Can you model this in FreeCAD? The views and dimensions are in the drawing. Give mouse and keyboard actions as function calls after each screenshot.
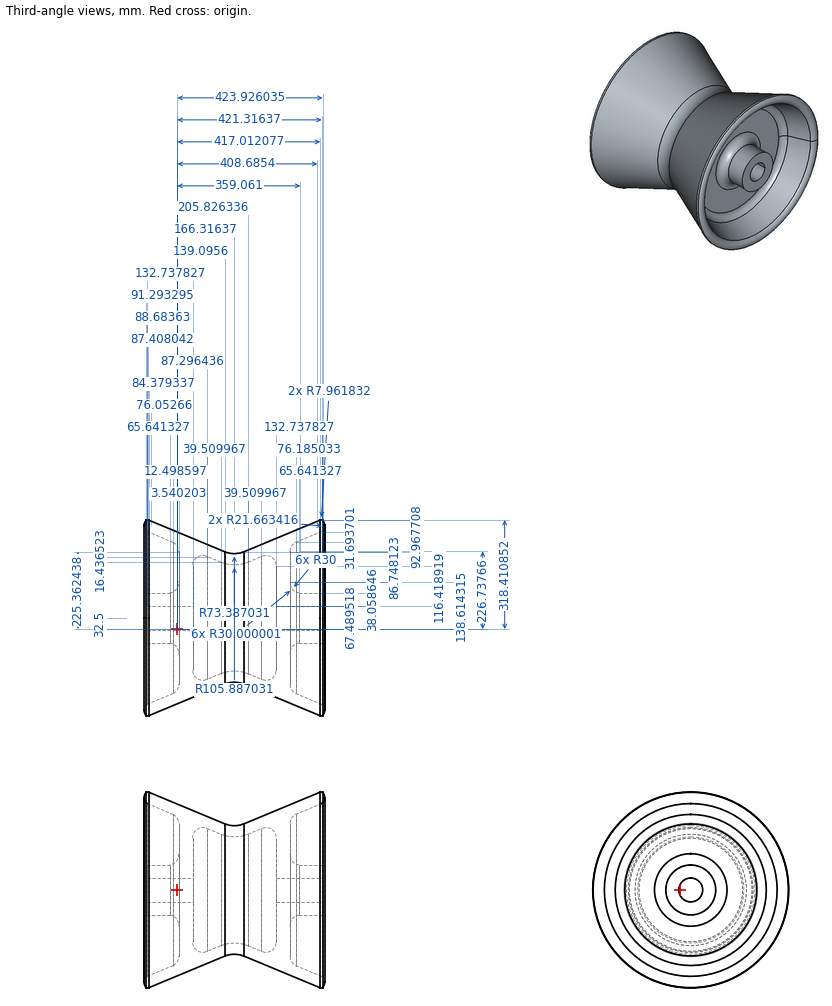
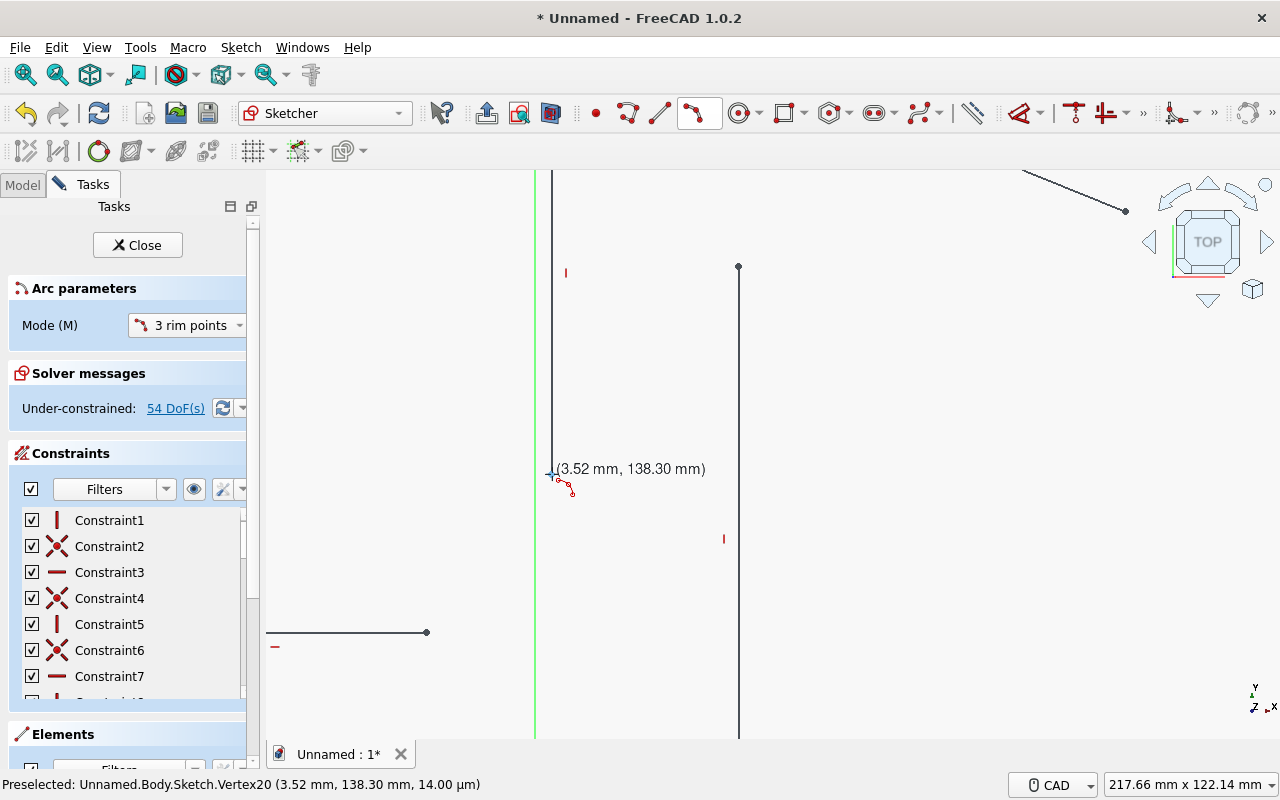
scroll(551, 474, down, 8)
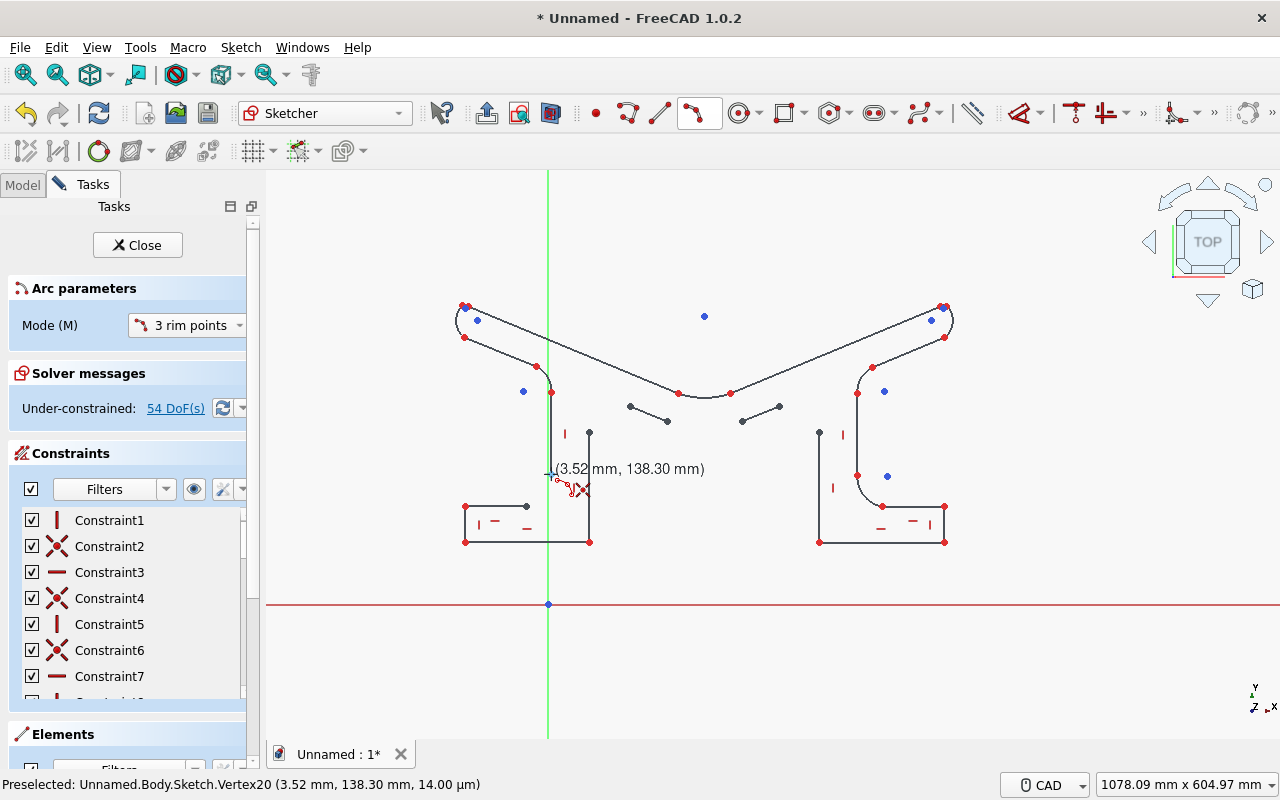
click(526, 506)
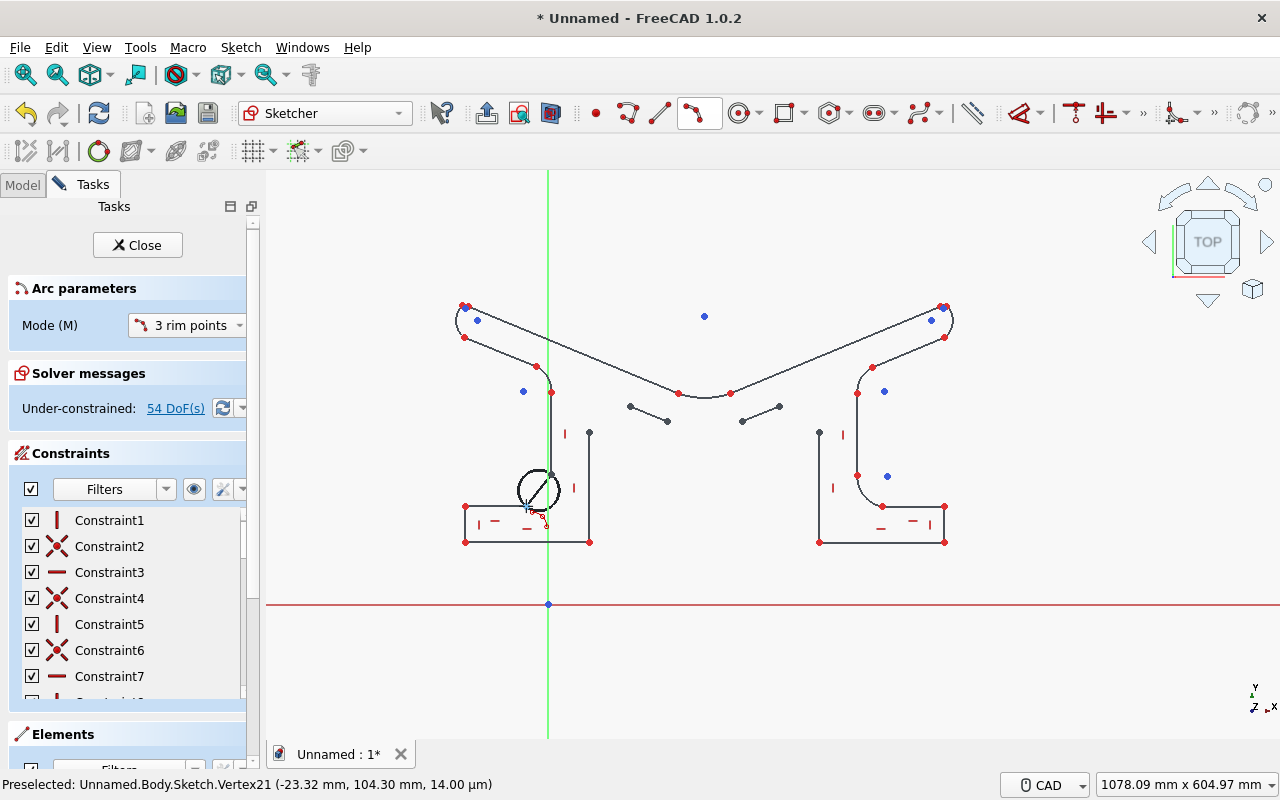
scroll(539, 501, up, 5)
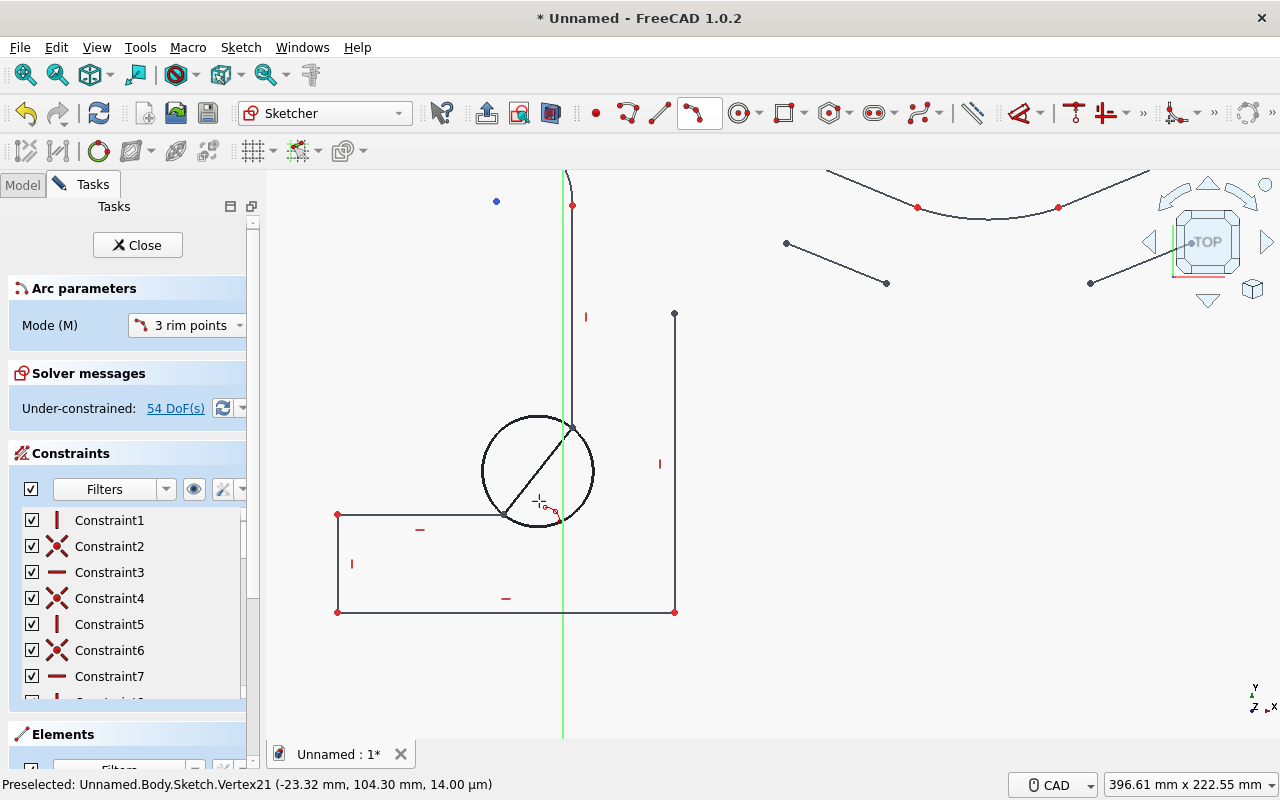
click(538, 500)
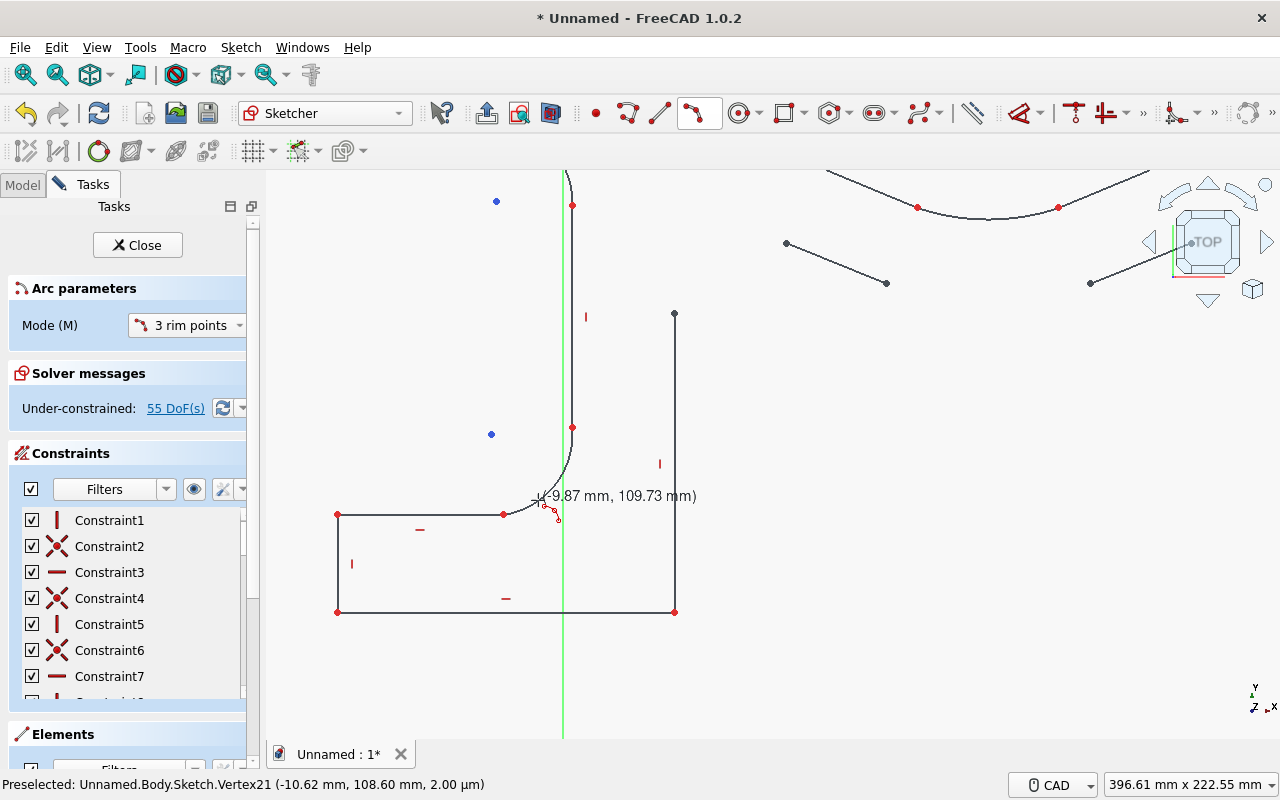
click(675, 314)
click(786, 243)
click(711, 244)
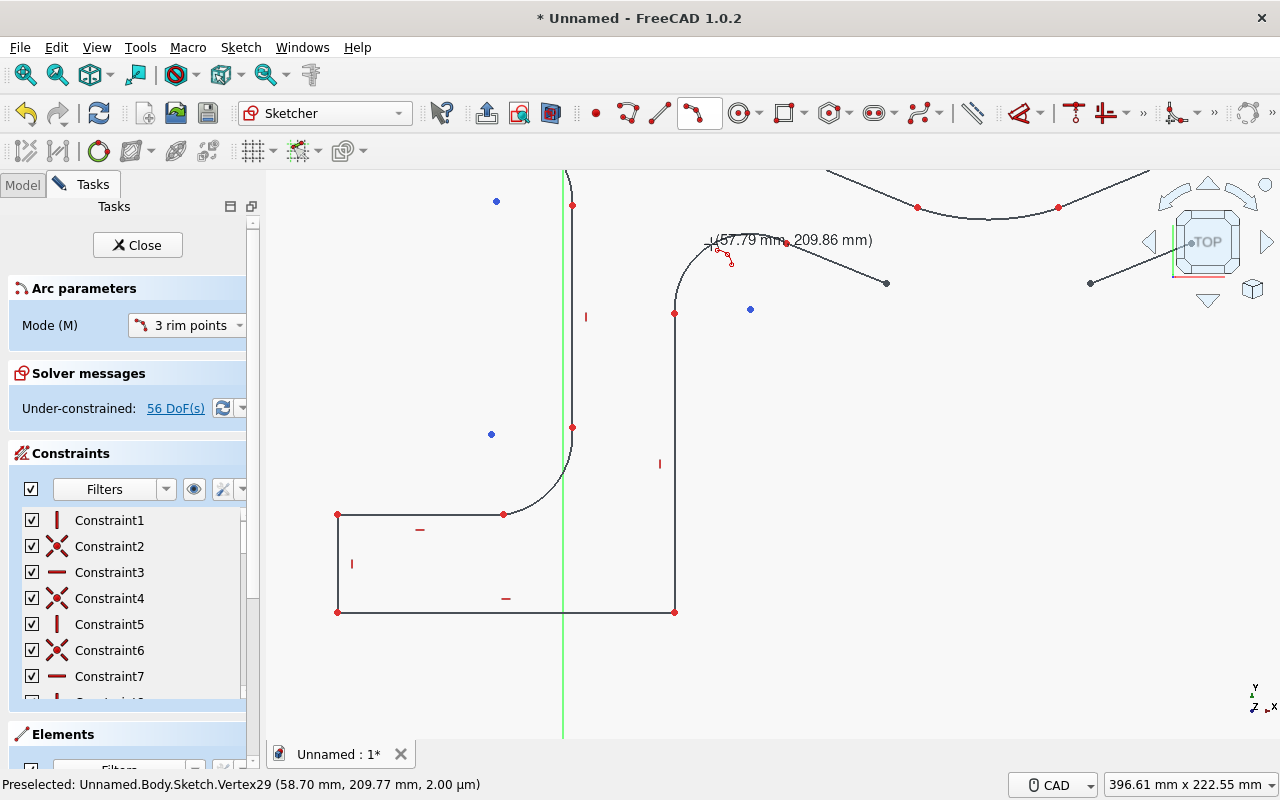
click(887, 284)
click(1091, 284)
click(988, 302)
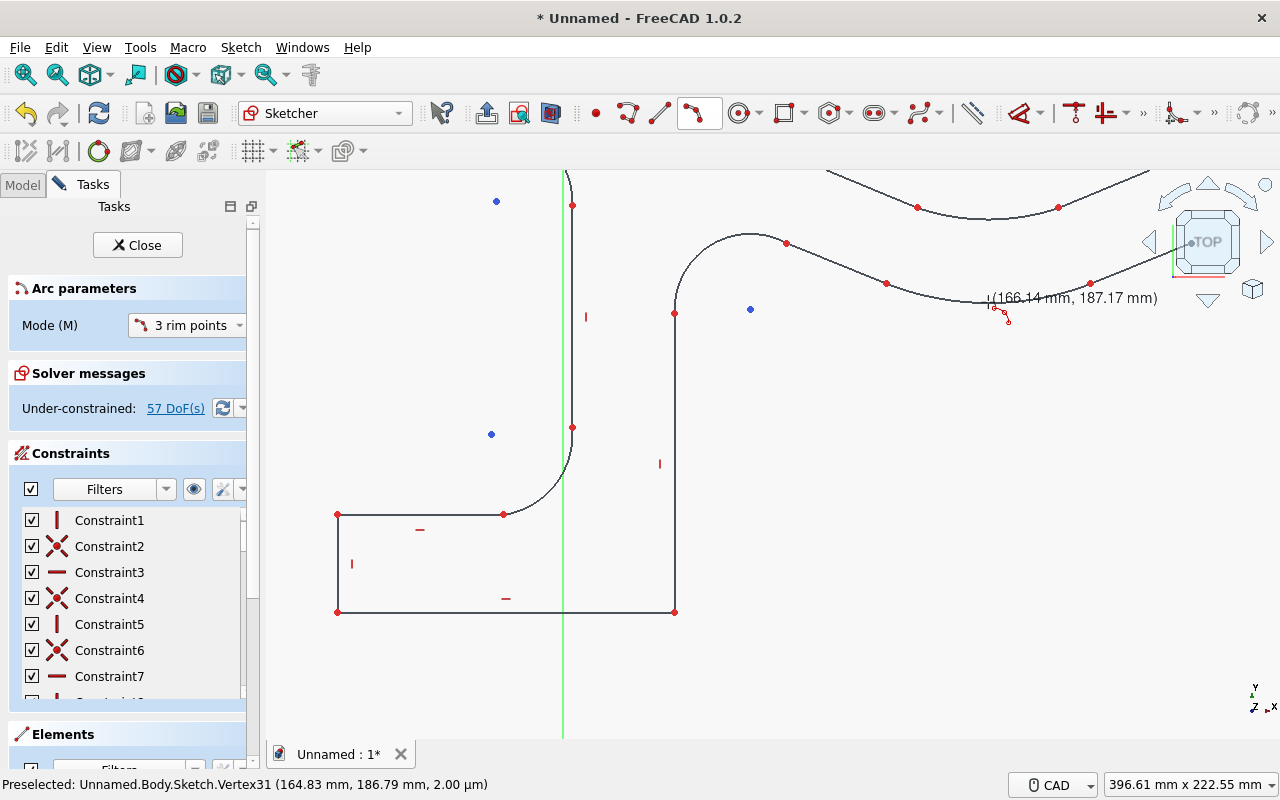
scroll(539, 501, down, 5)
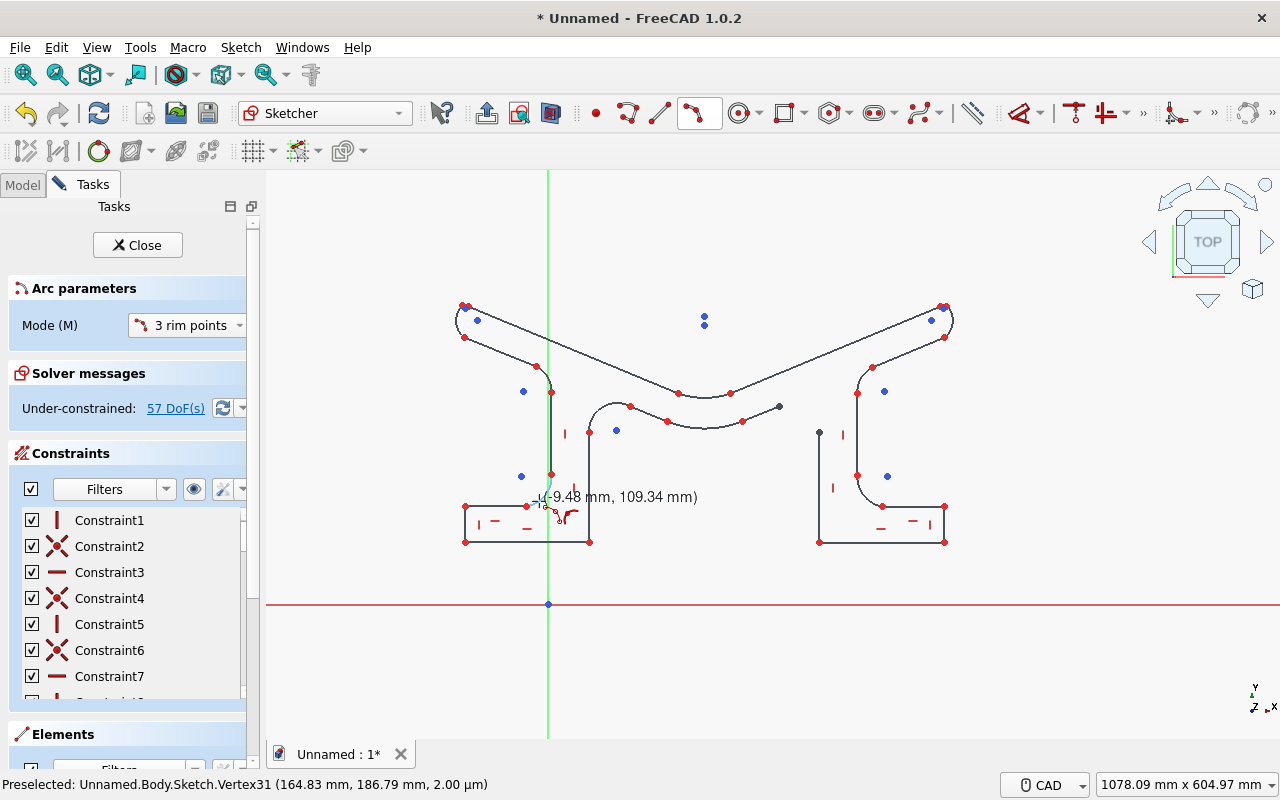
click(779, 406)
click(819, 433)
click(807, 407)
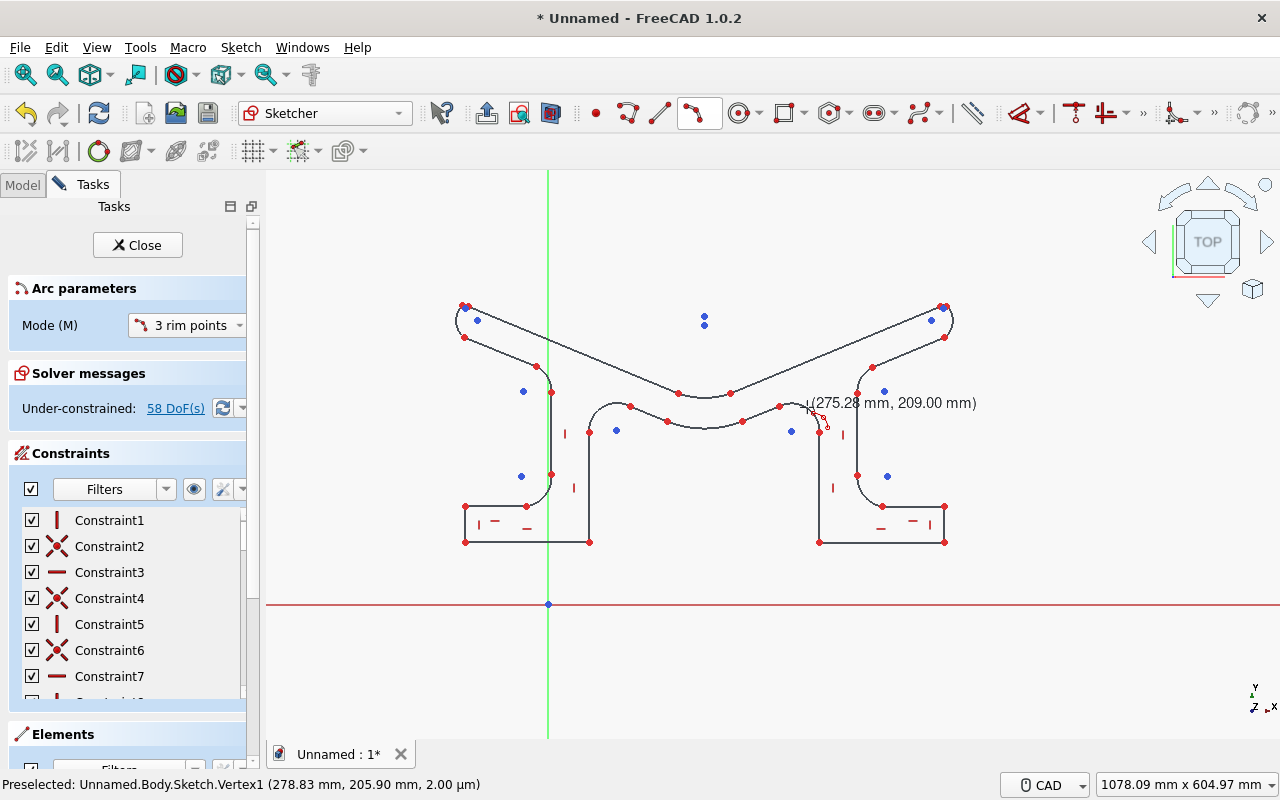
click(660, 114)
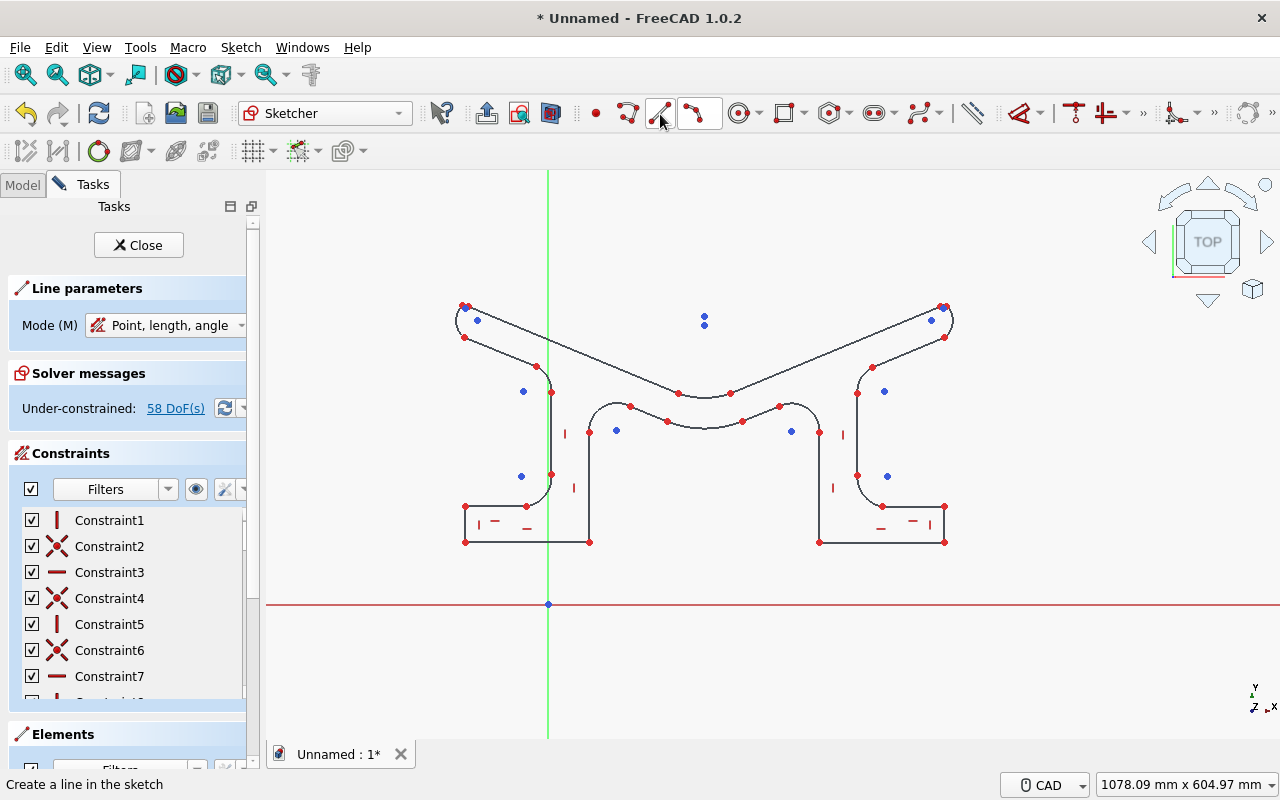
click(407, 574)
click(1002, 574)
key(Escape)